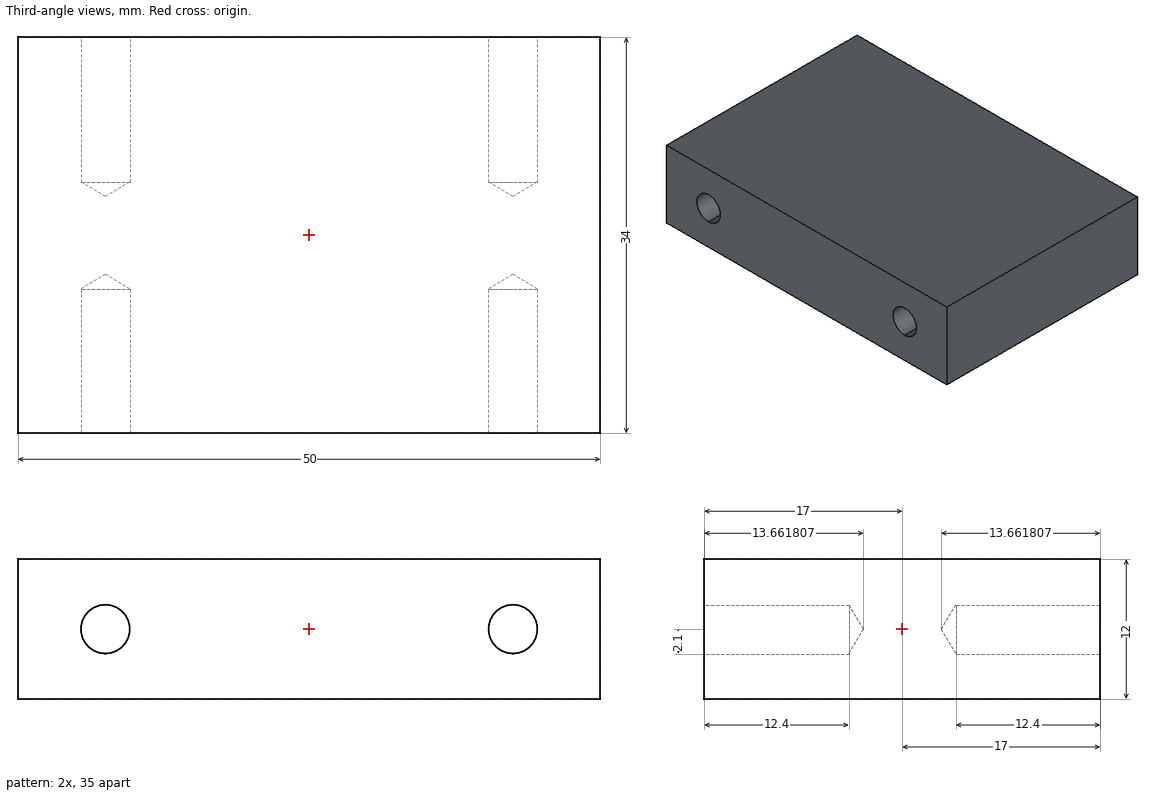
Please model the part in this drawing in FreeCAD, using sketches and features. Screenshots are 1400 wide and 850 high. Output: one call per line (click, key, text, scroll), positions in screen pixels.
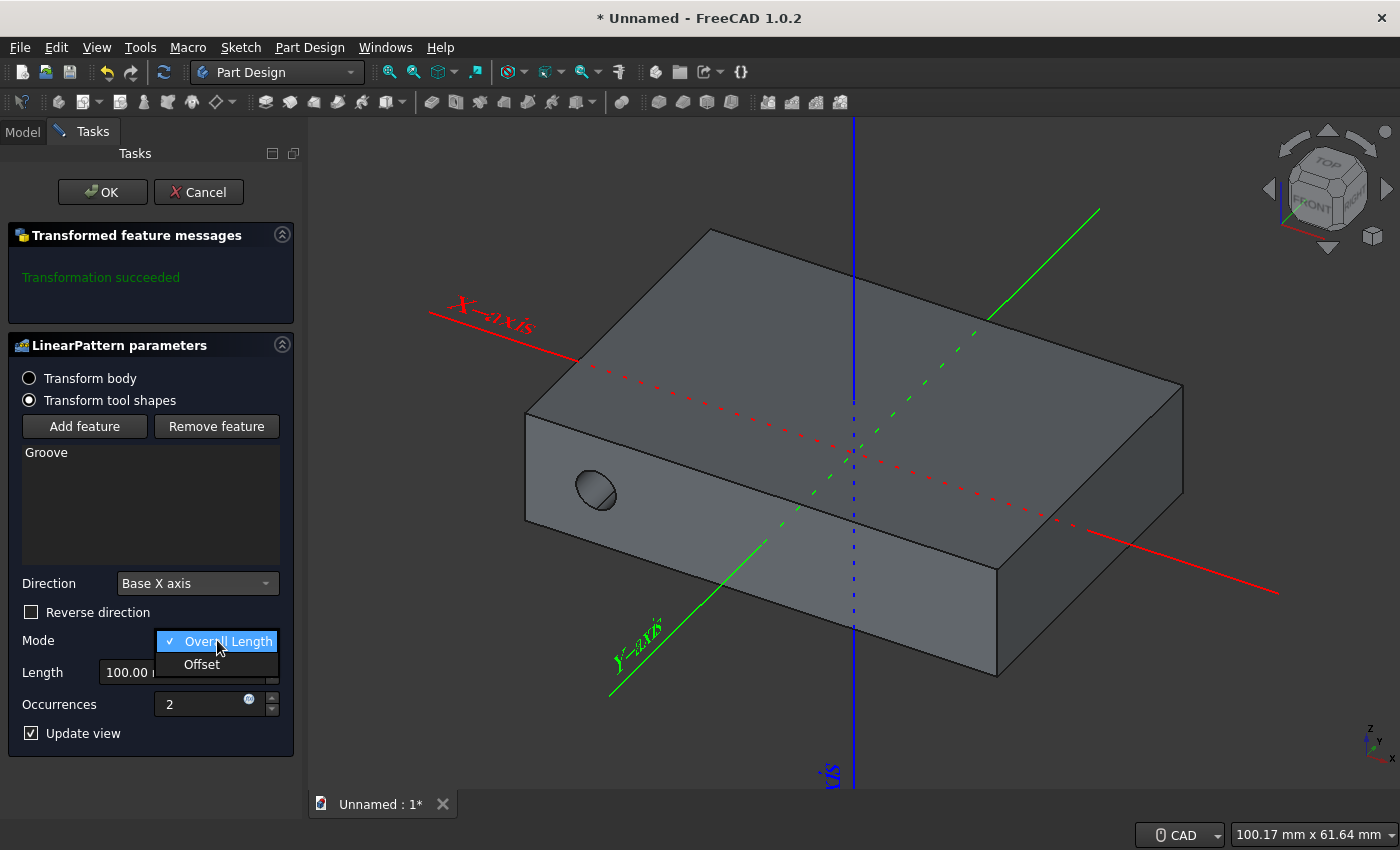
click(216, 664)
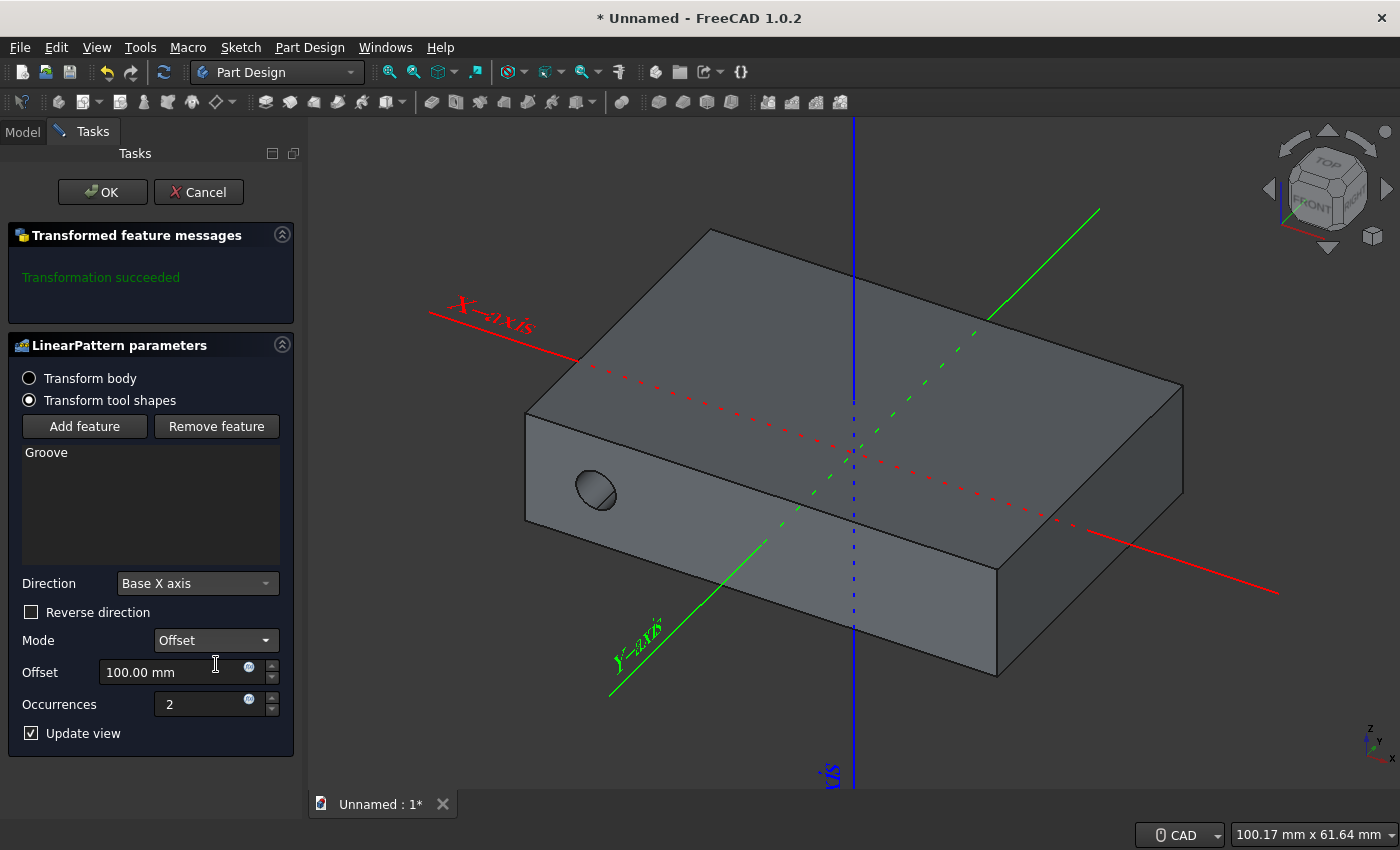
triple_click(182, 672)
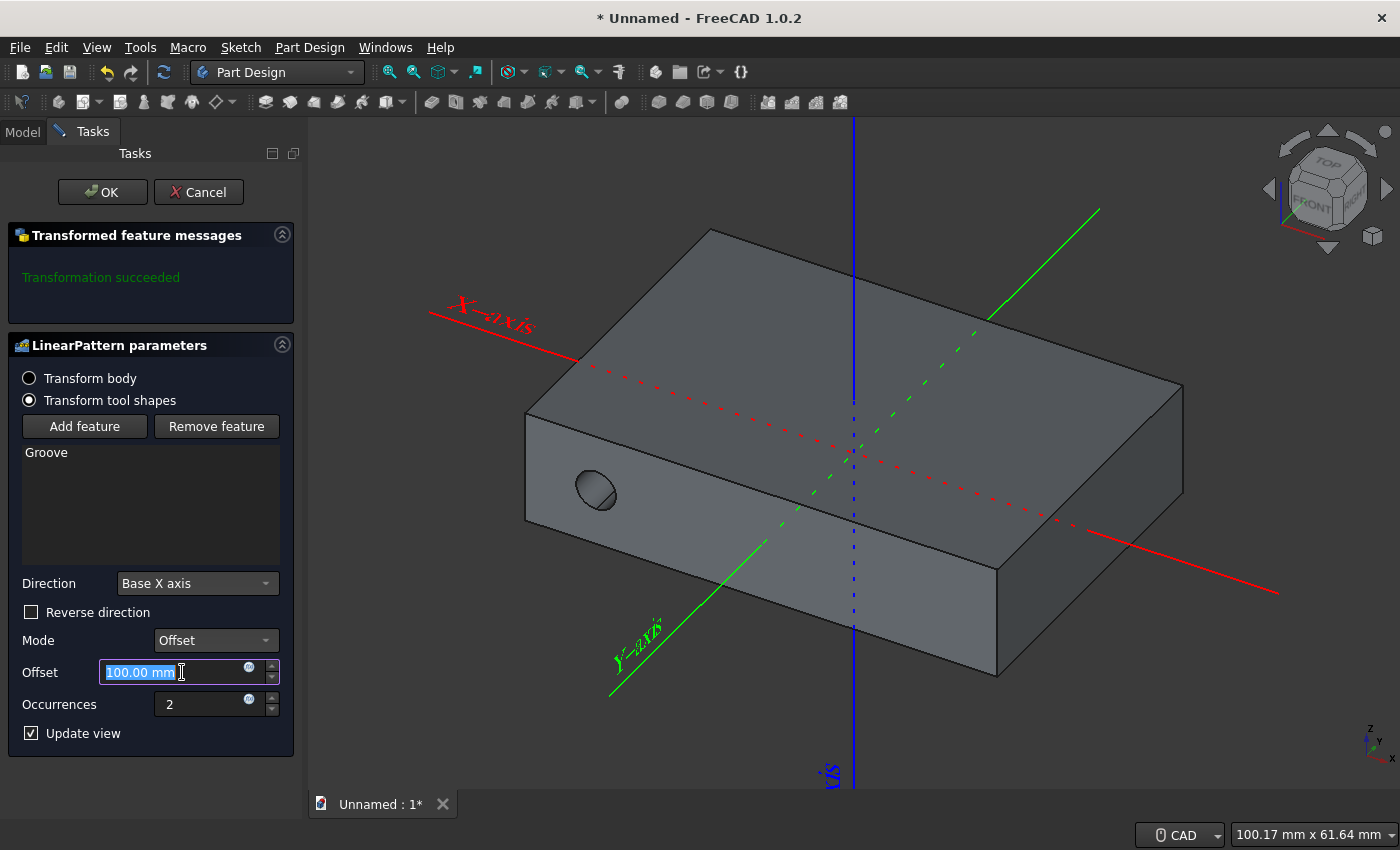
text(35)
key(Tab)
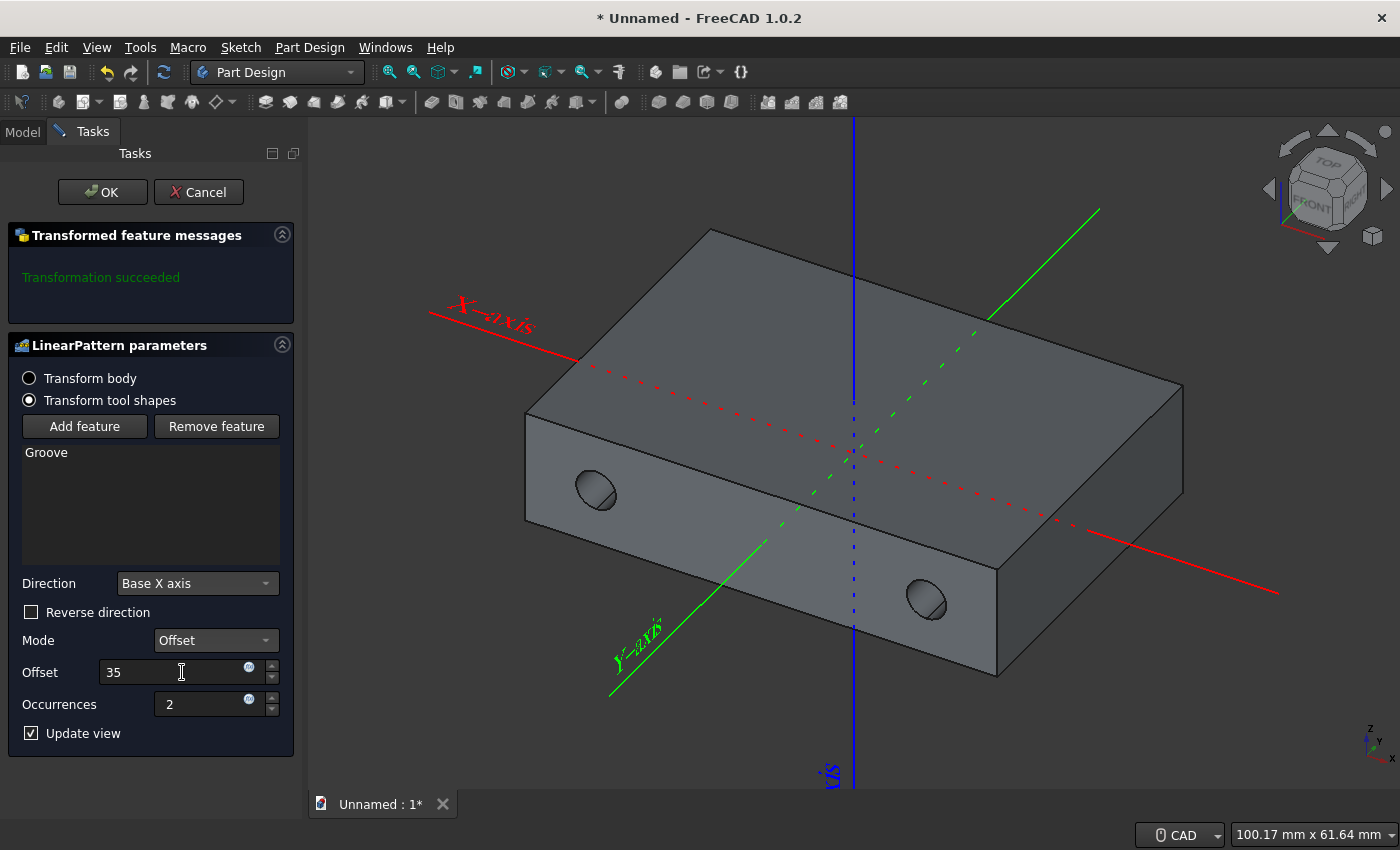
triple_click(209, 704)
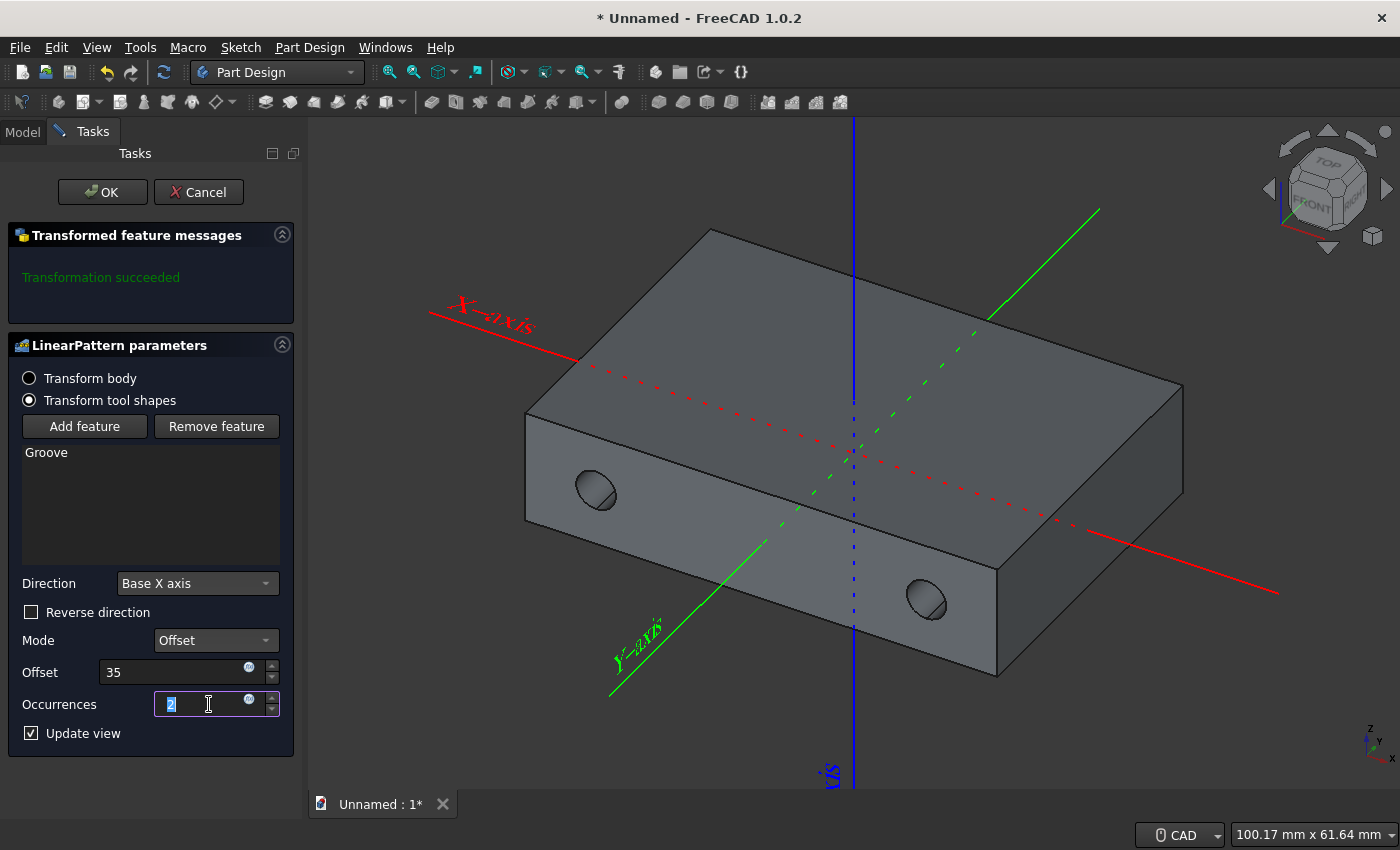
text(2)
key(Tab)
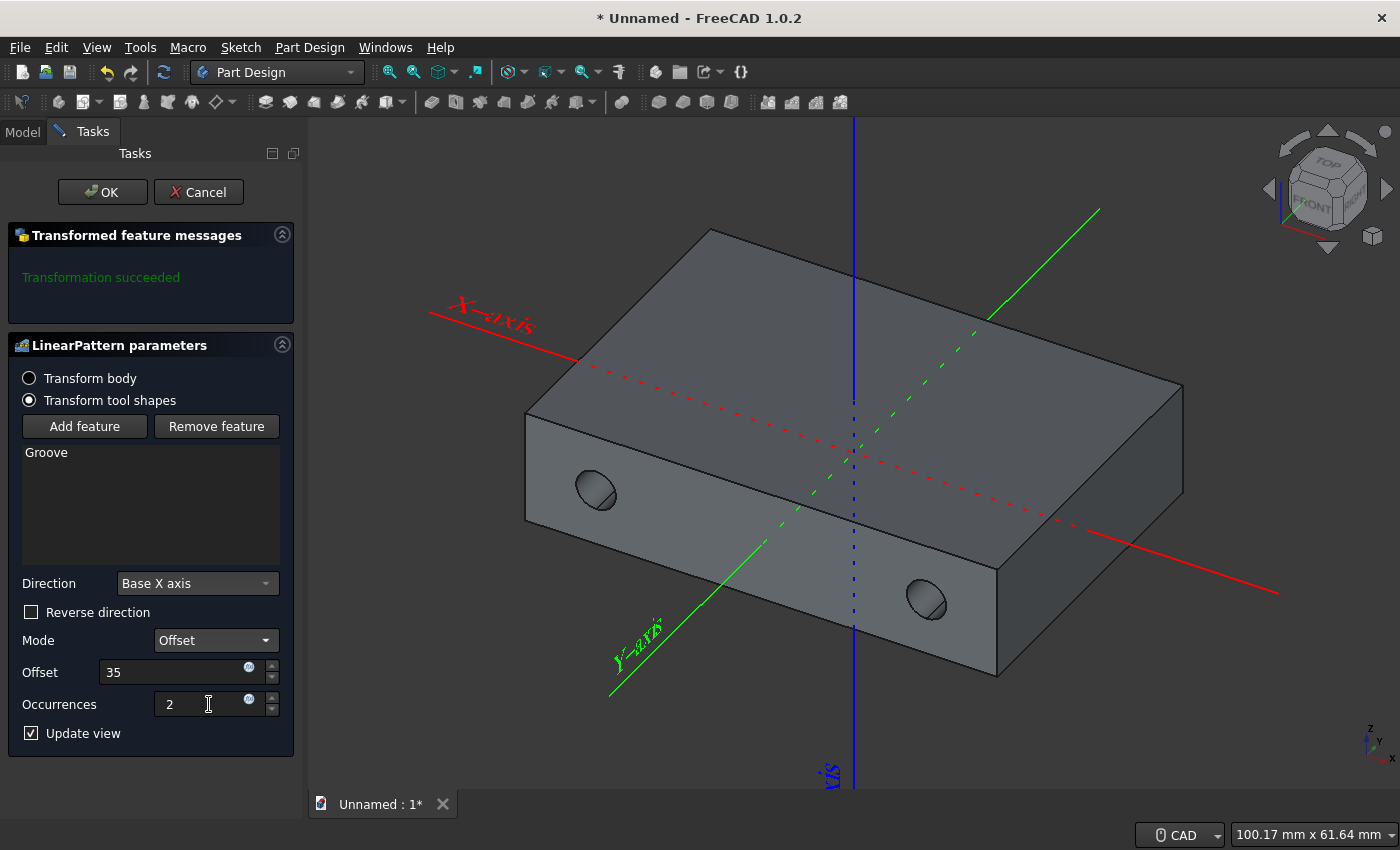
click(103, 192)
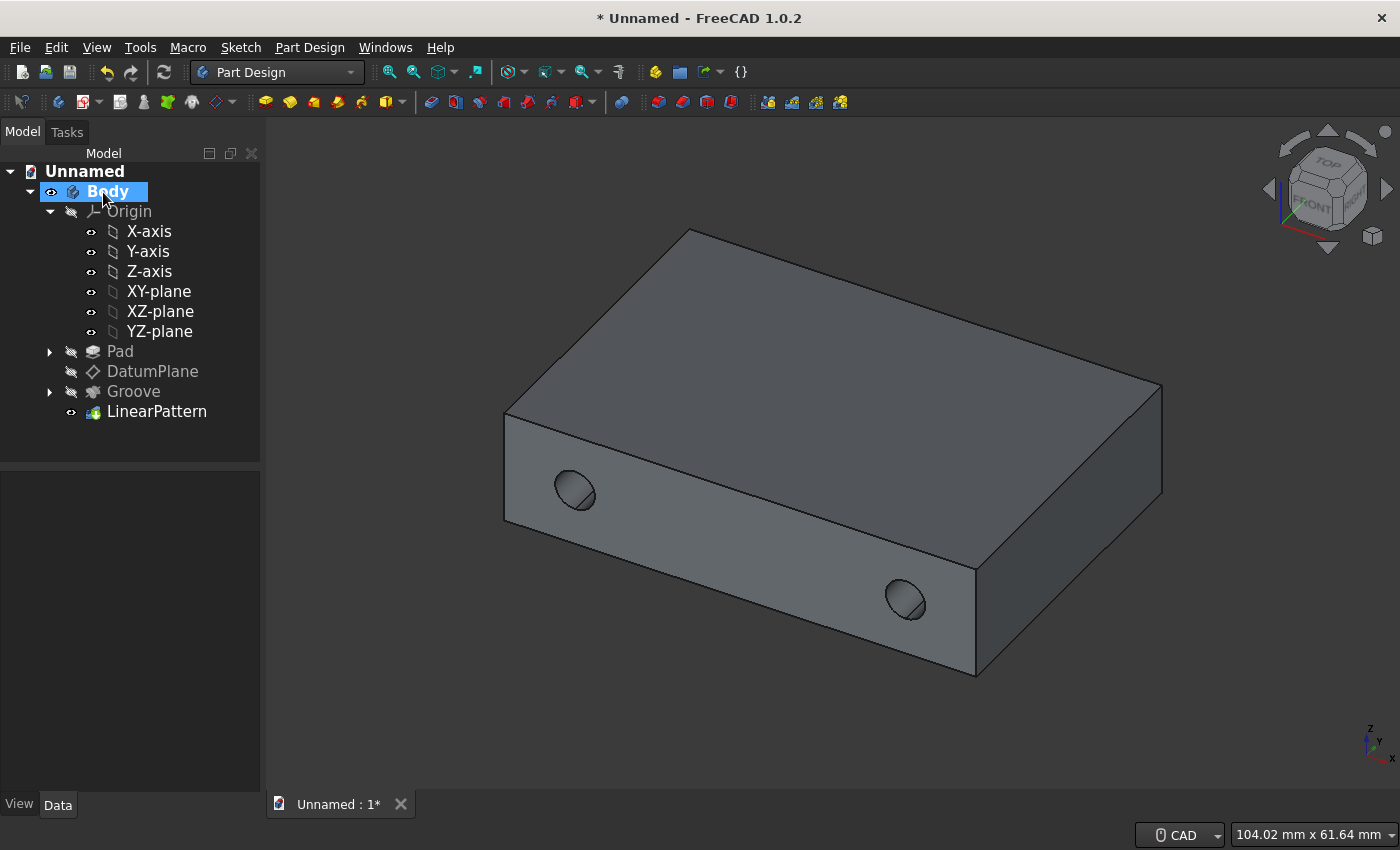
click(116, 392)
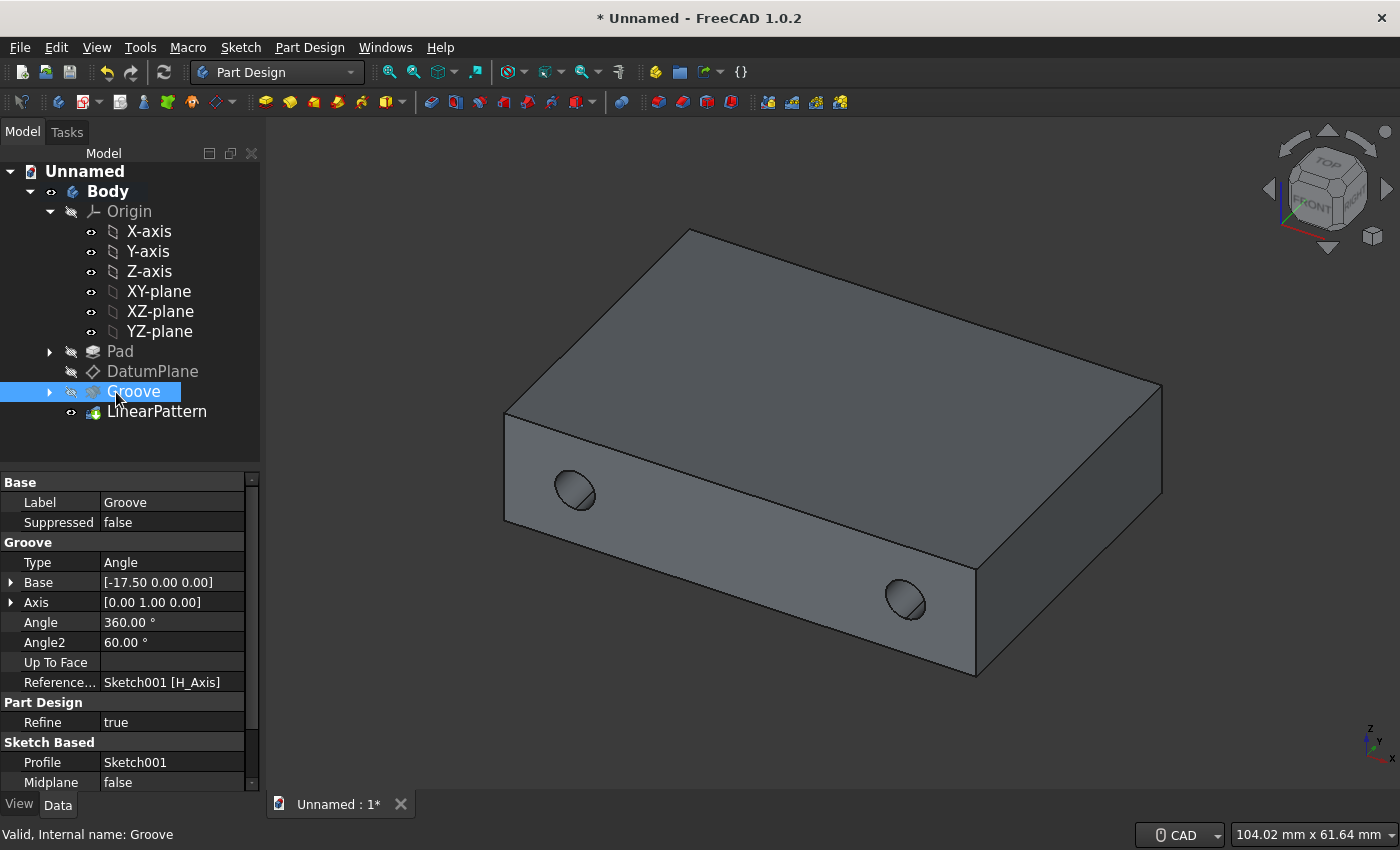
click(768, 102)